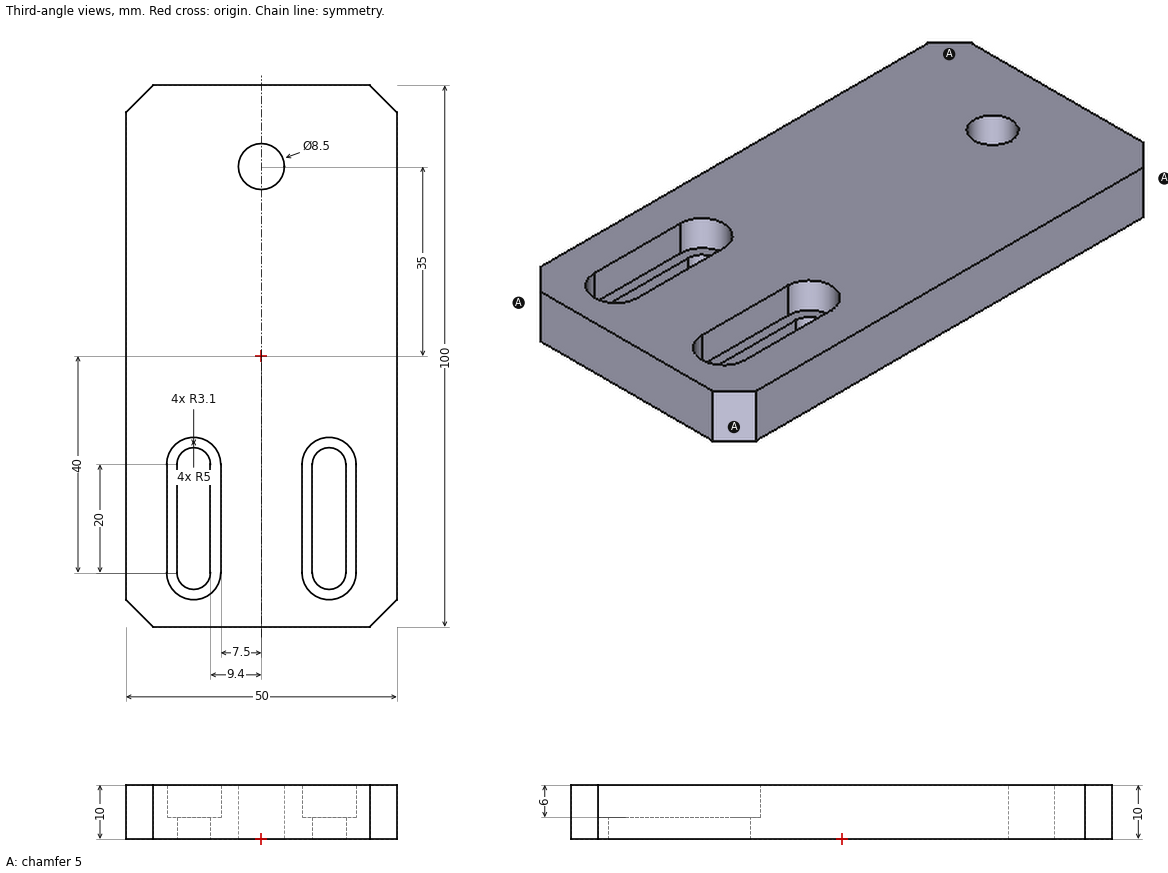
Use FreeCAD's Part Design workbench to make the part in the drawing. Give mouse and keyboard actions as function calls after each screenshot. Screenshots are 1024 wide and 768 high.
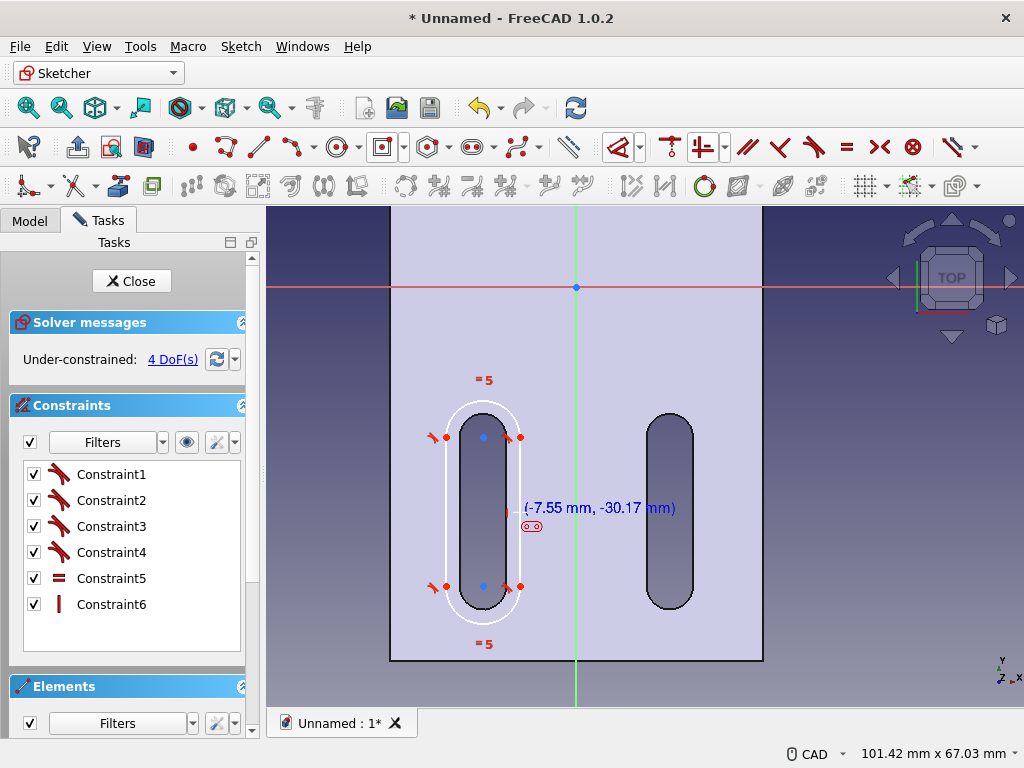
click(670, 586)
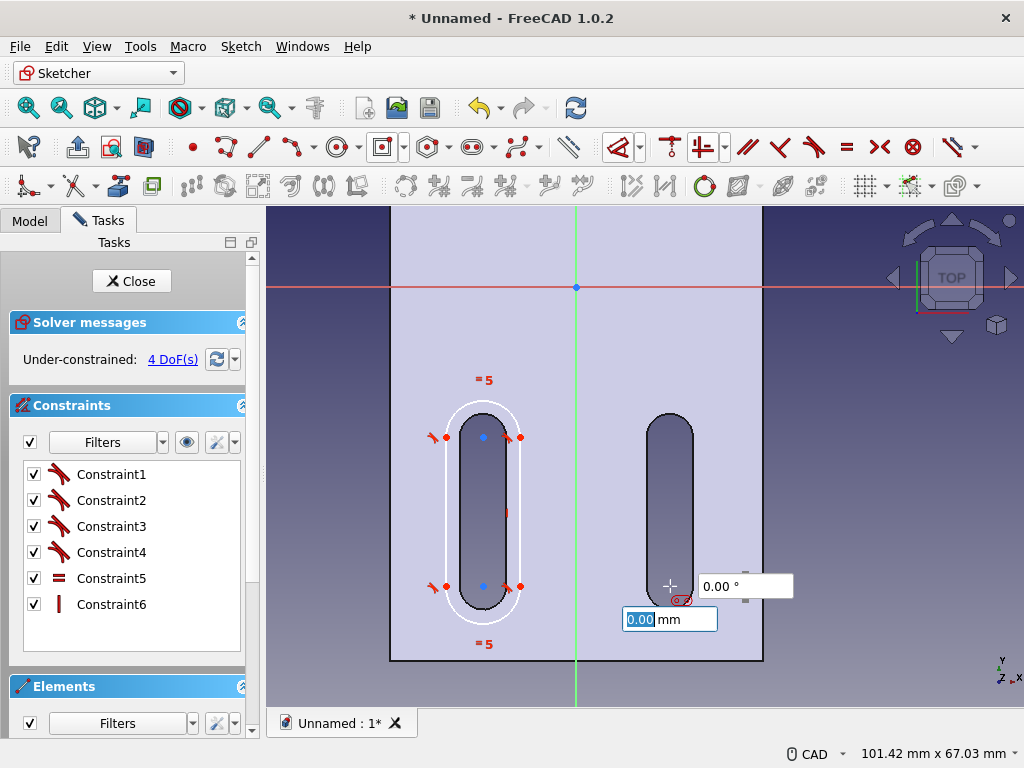
click(670, 437)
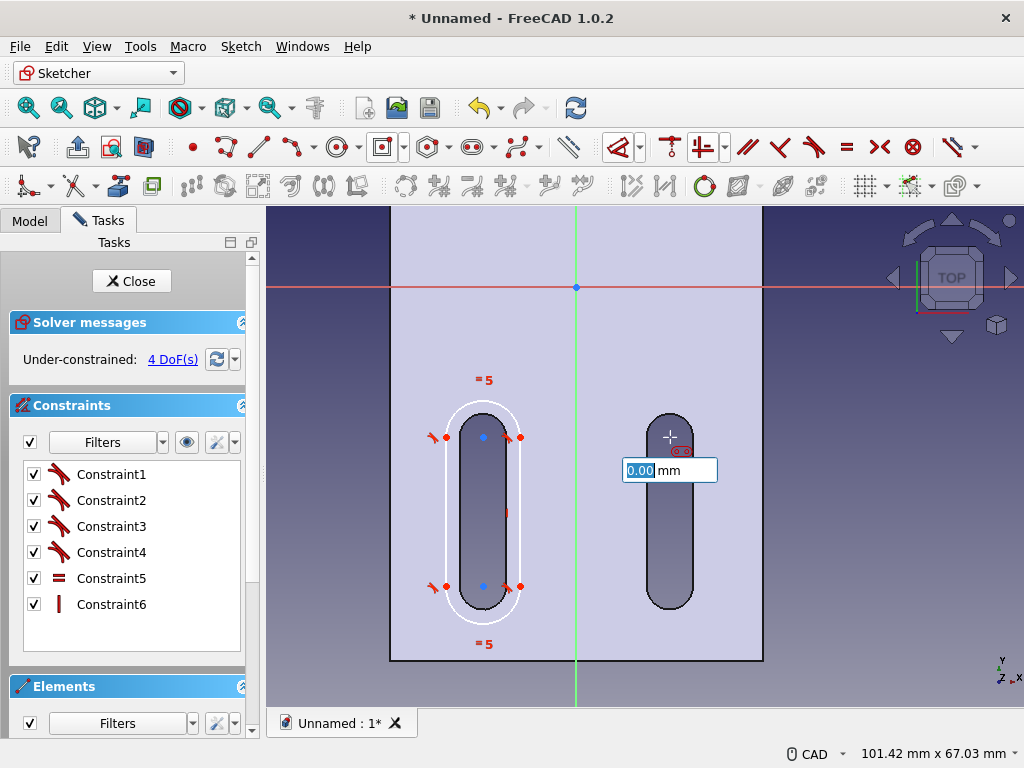
click(707, 512)
key(Escape)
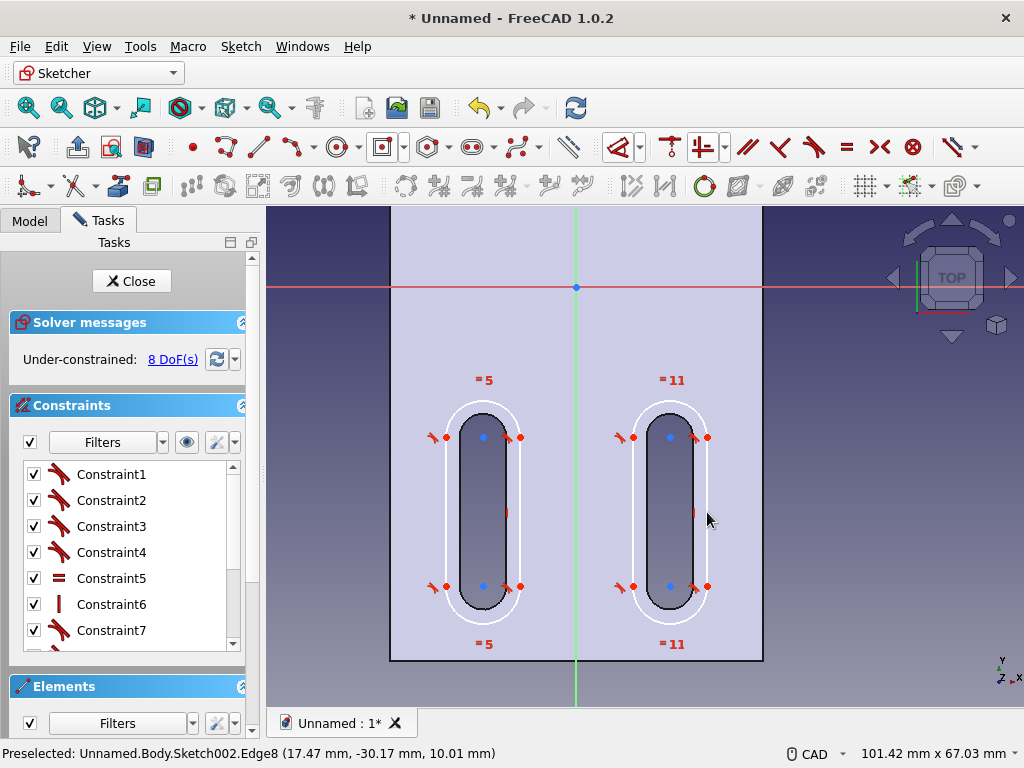
click(461, 617)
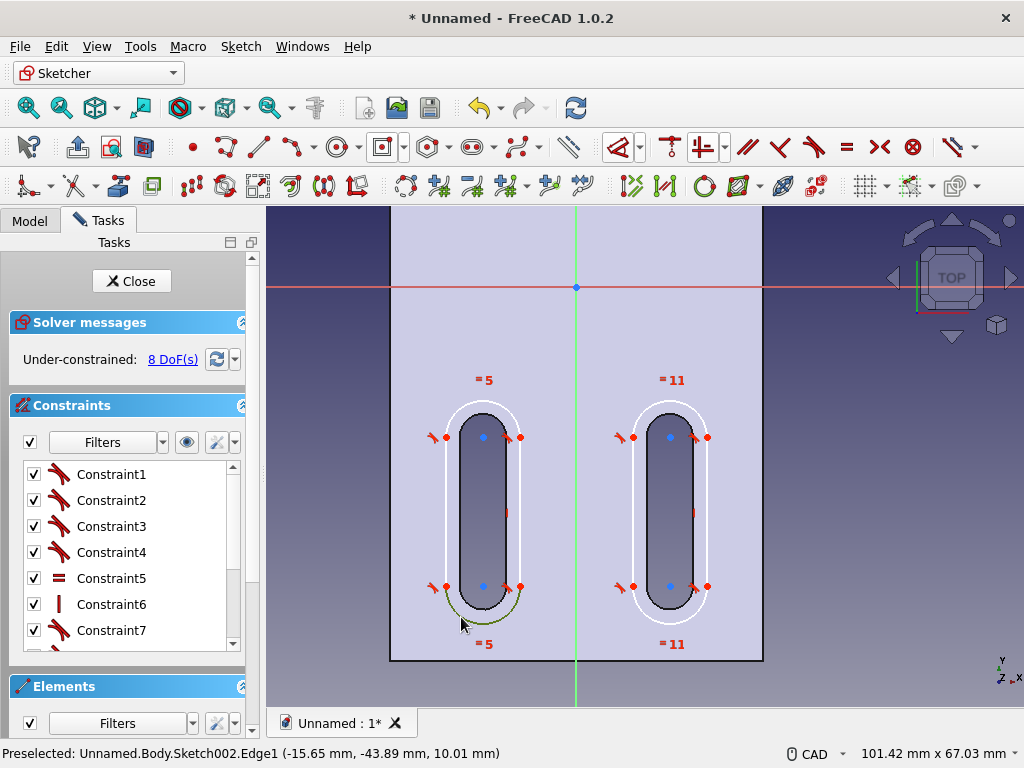
click(648, 617)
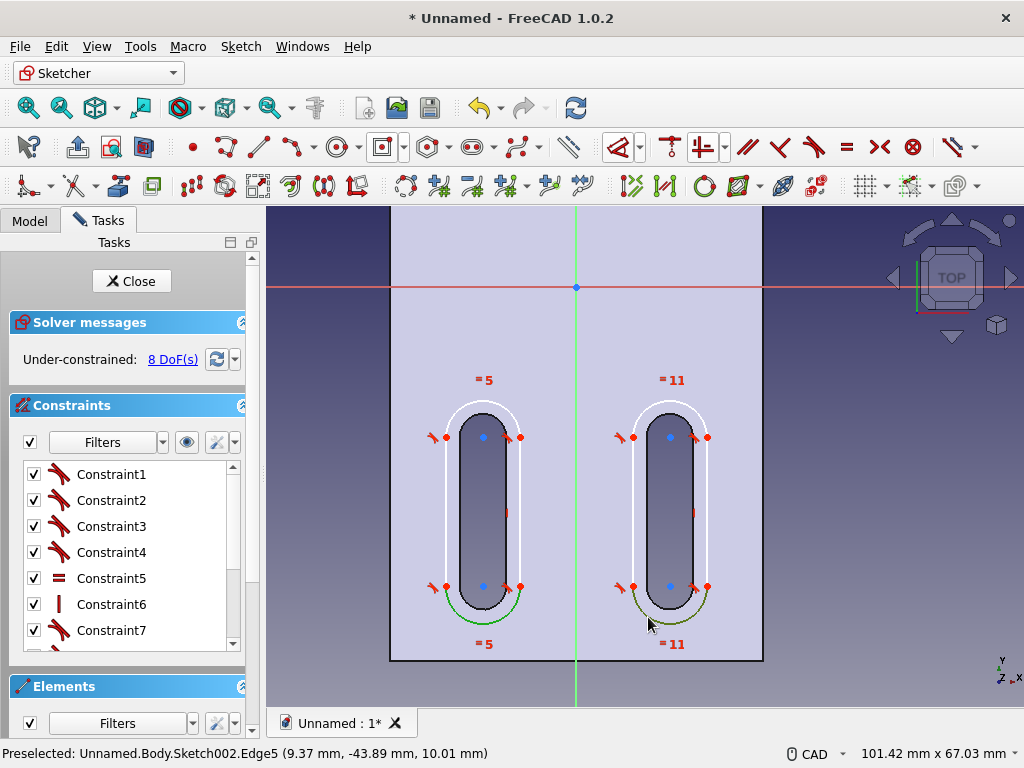
click(847, 148)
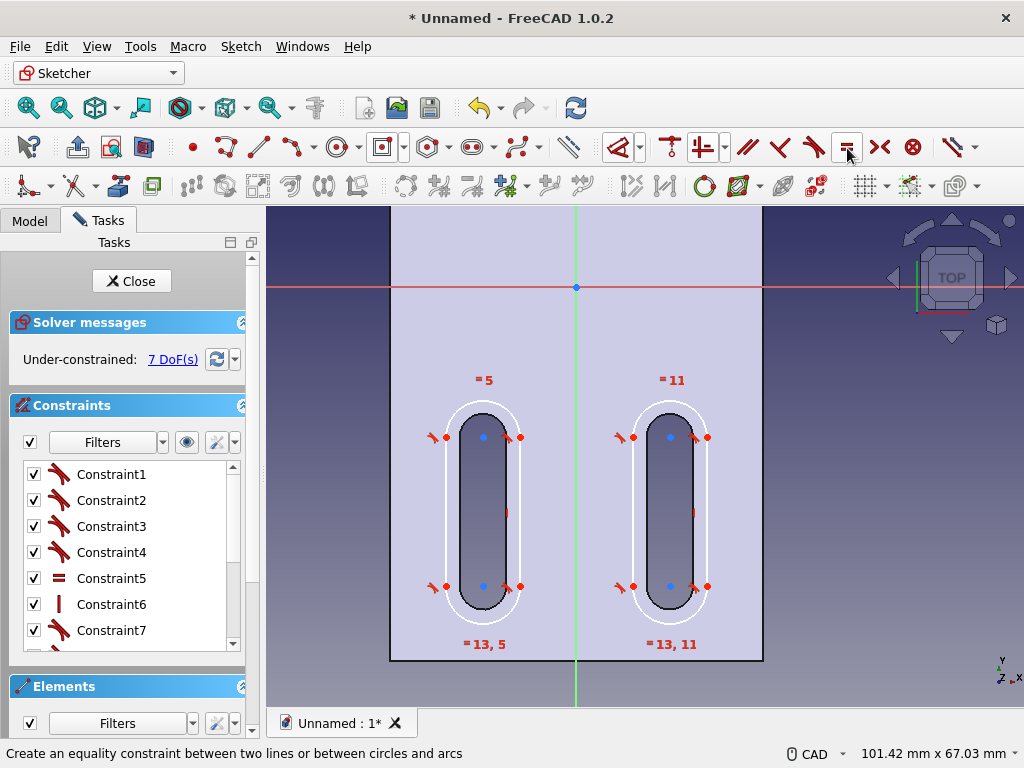
click(483, 587)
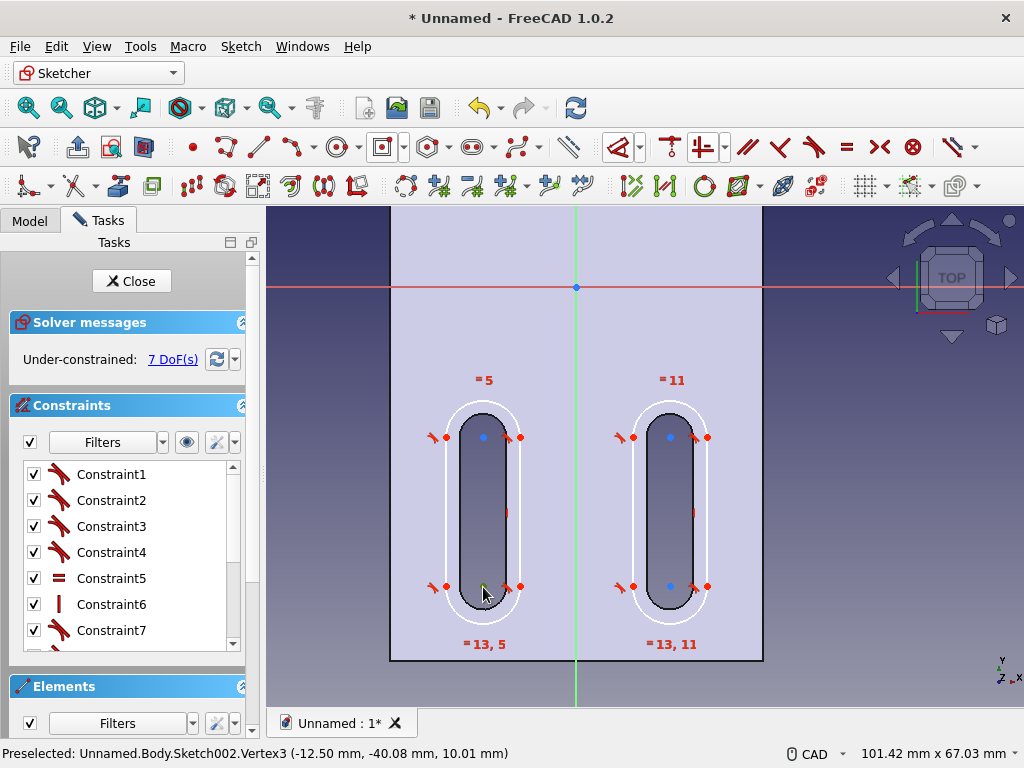
click(670, 587)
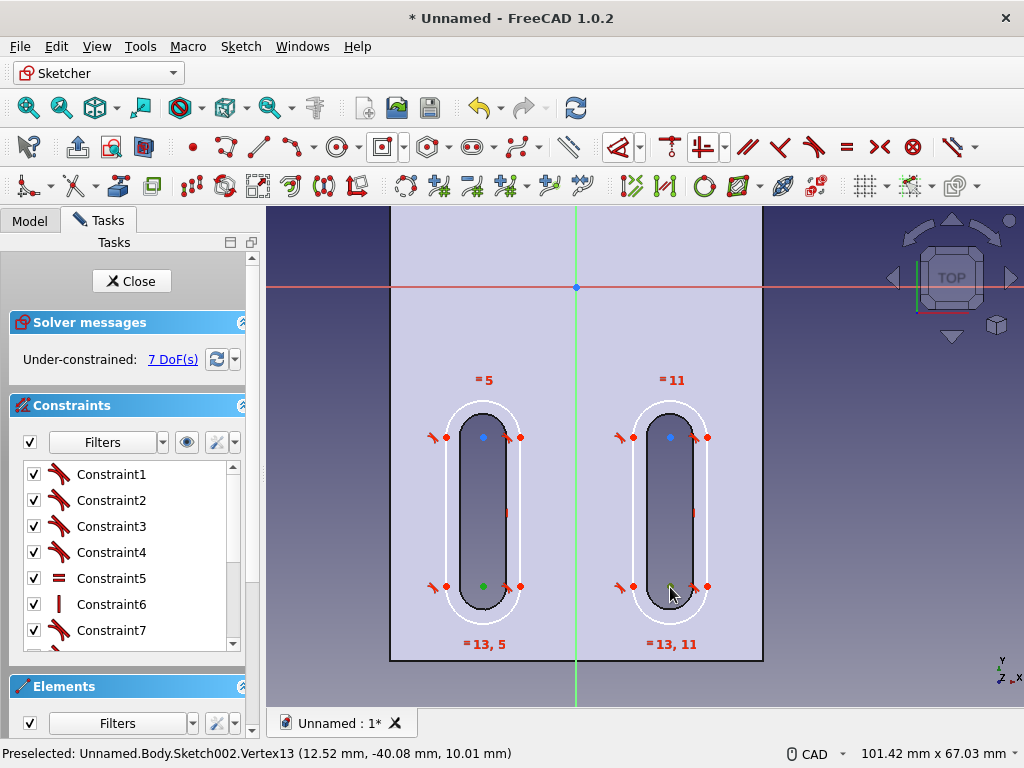
click(576, 647)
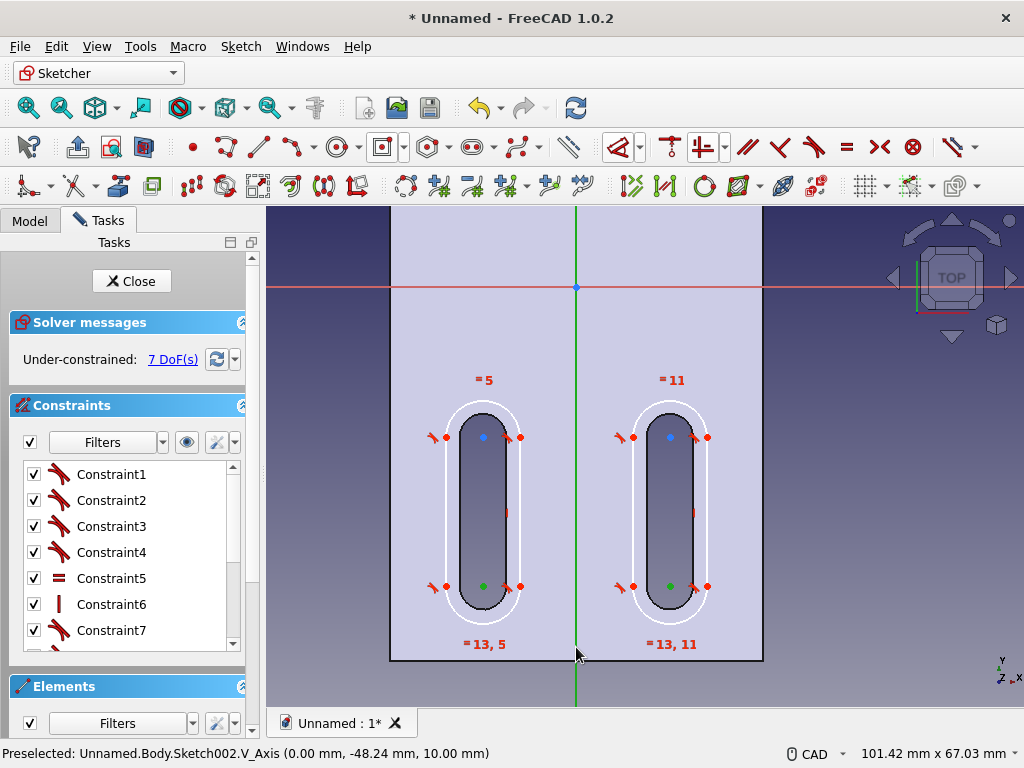
click(880, 148)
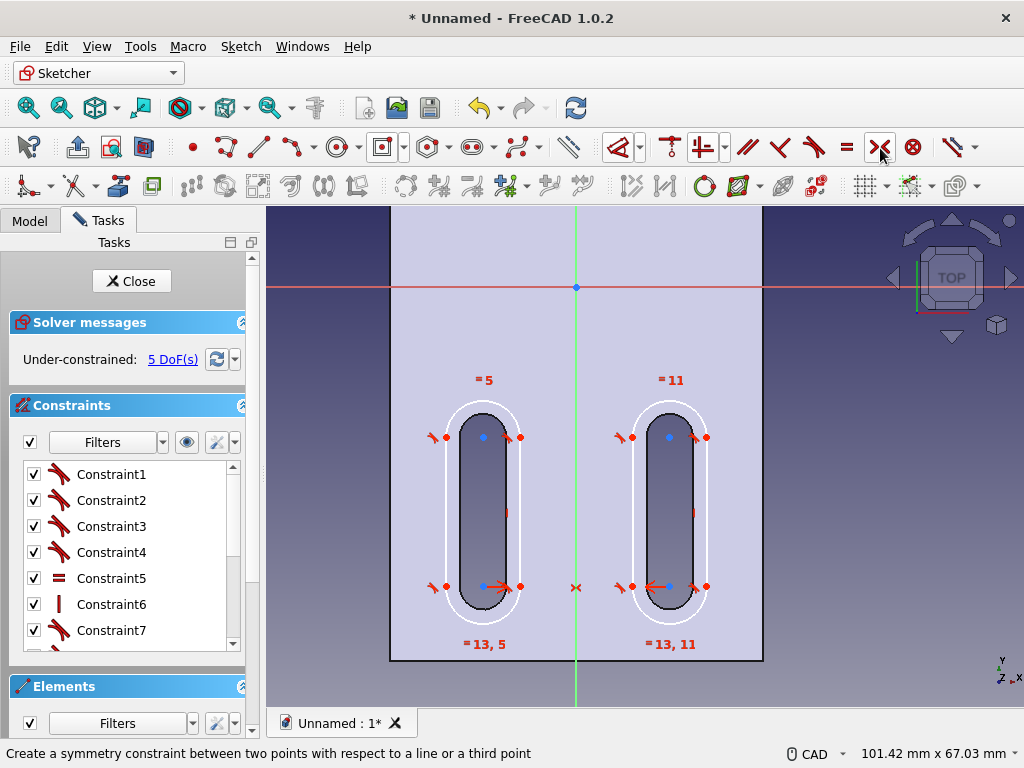
click(461, 617)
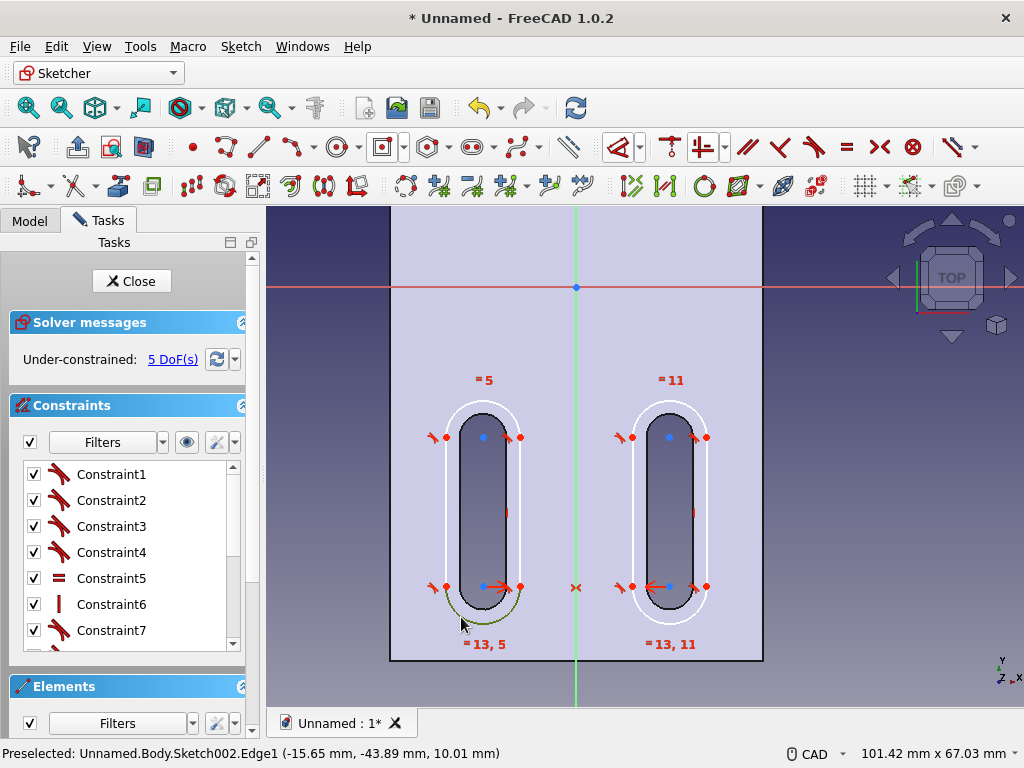
click(640, 148)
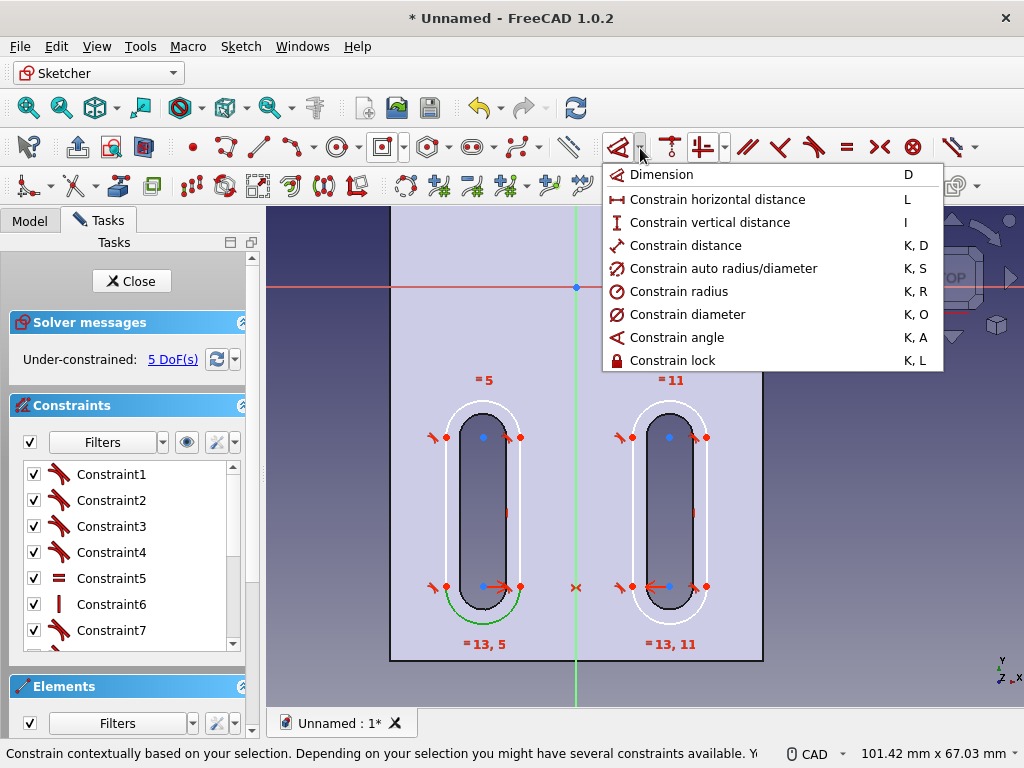
click(773, 292)